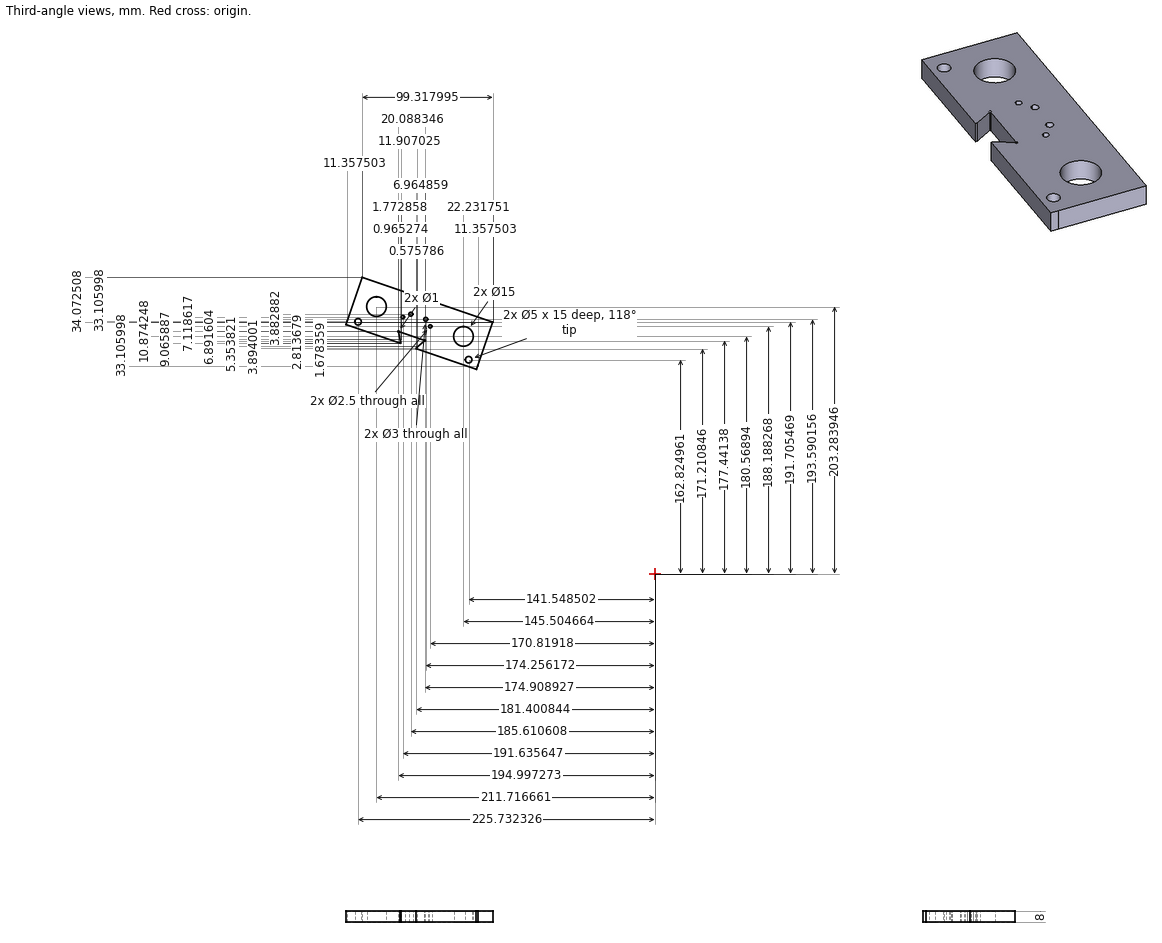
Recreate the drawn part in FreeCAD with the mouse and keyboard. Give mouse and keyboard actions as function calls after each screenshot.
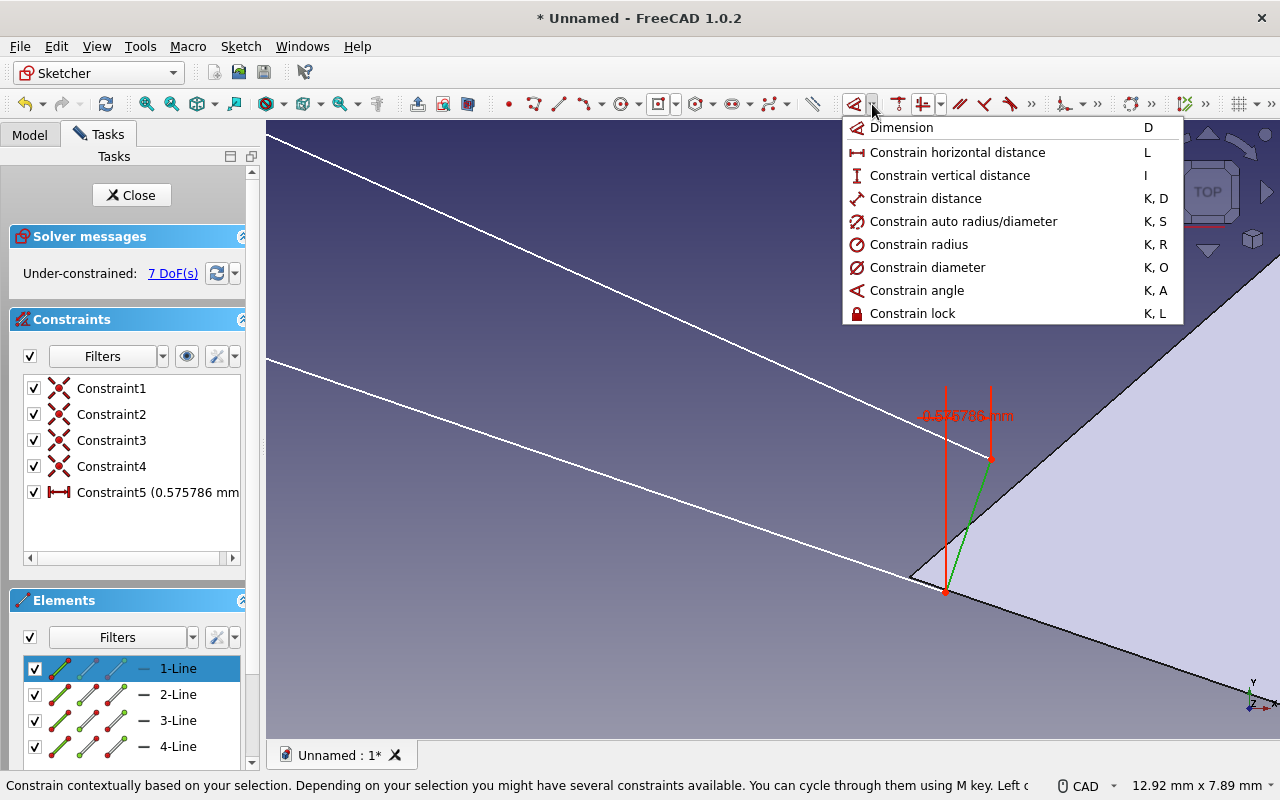
click(1013, 176)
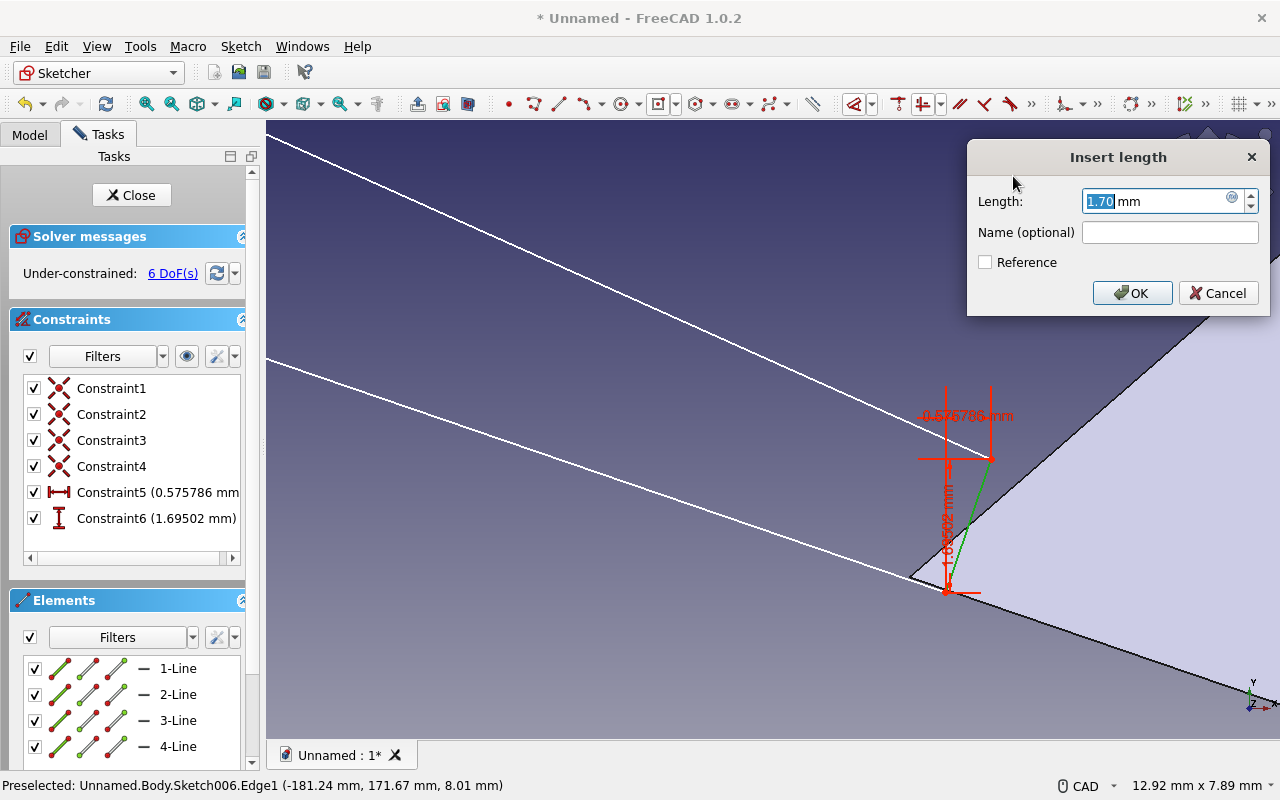
text(1.678359)
key(Return)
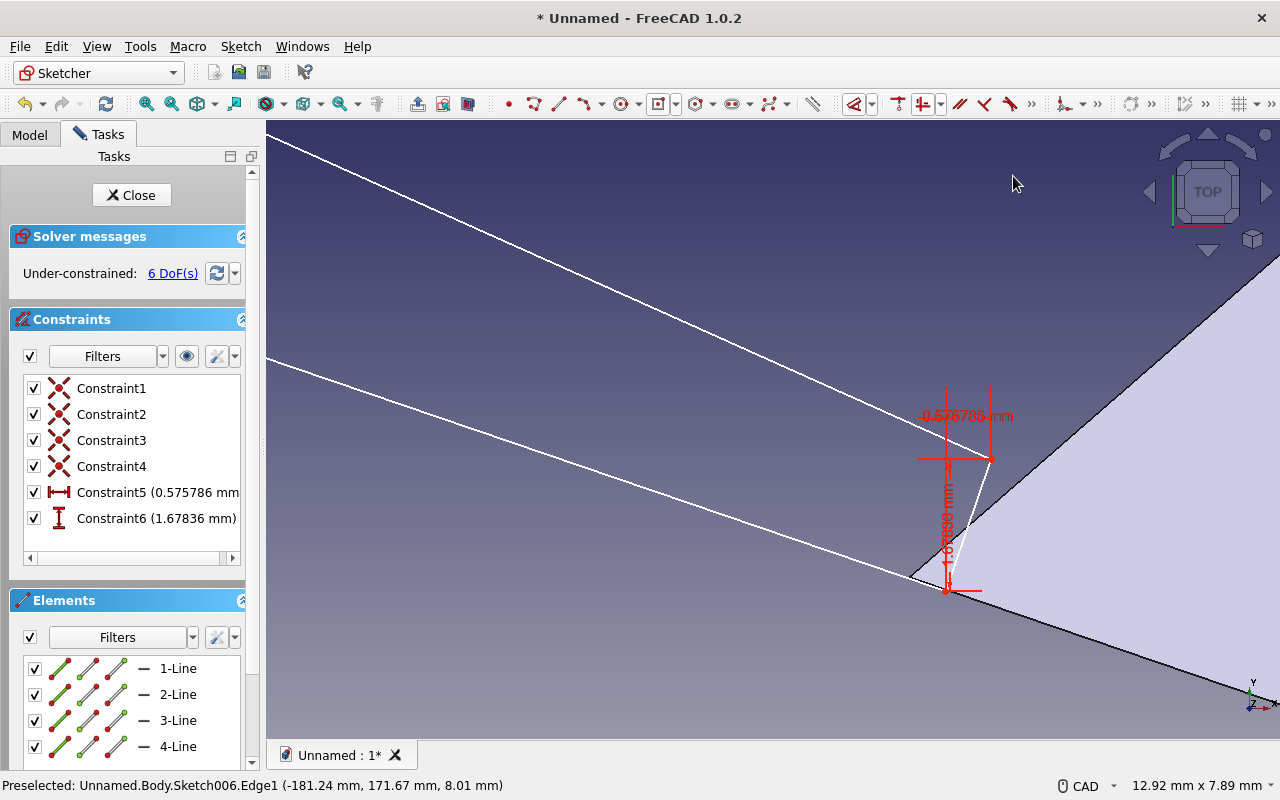
click(711, 334)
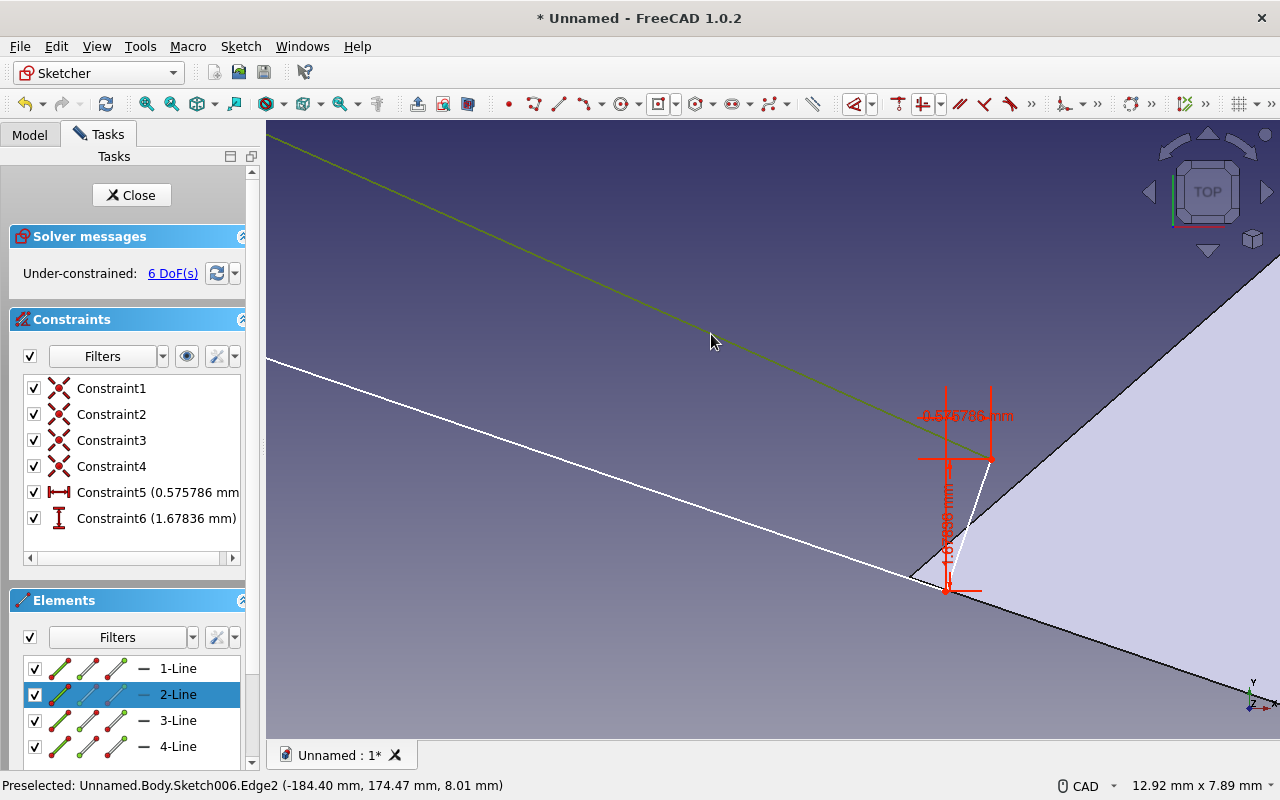
click(872, 104)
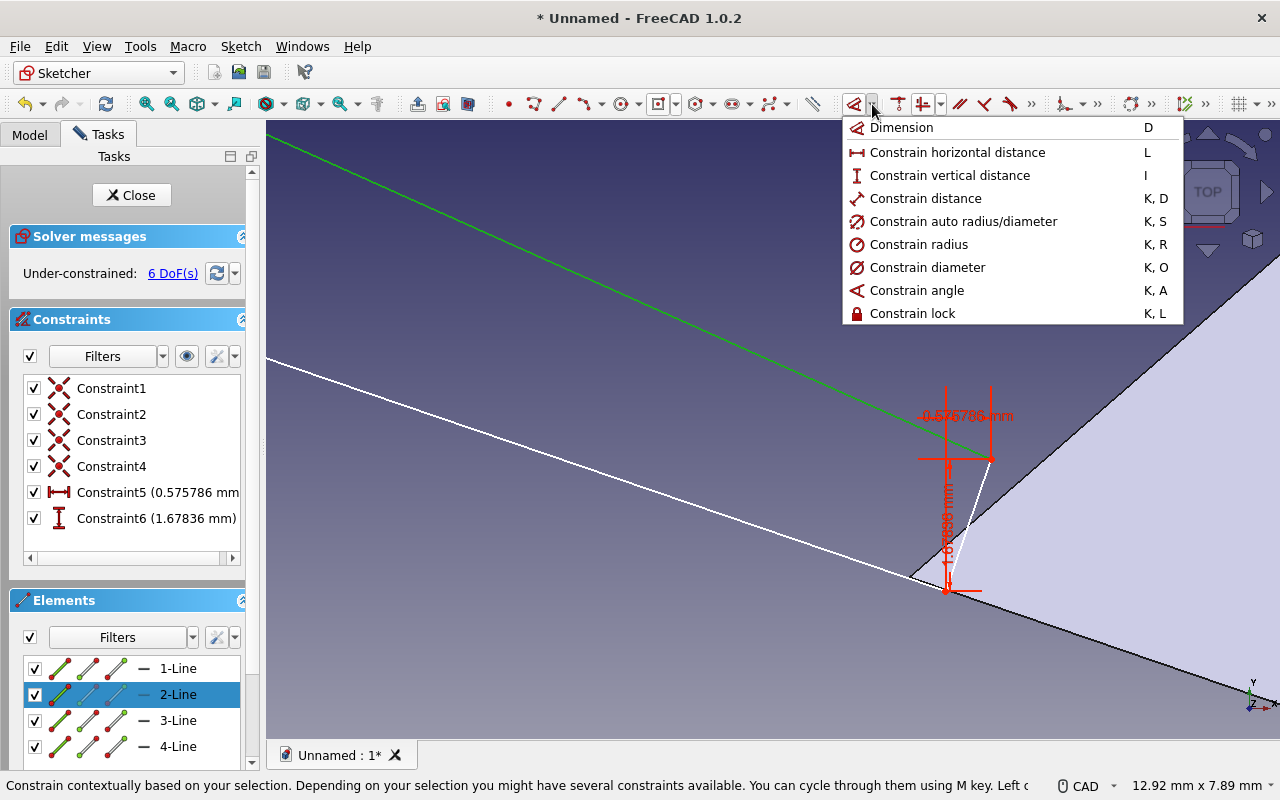
click(1013, 176)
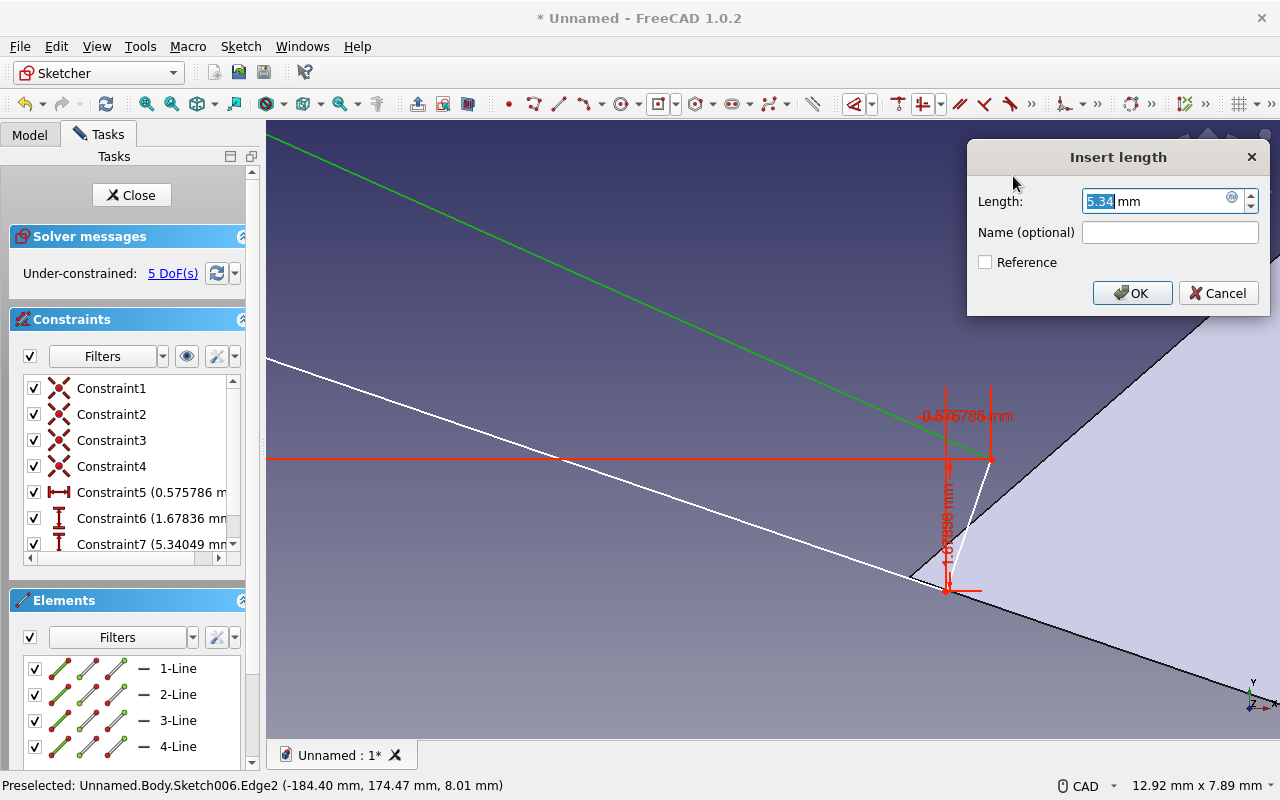
text(5.353821)
key(Return)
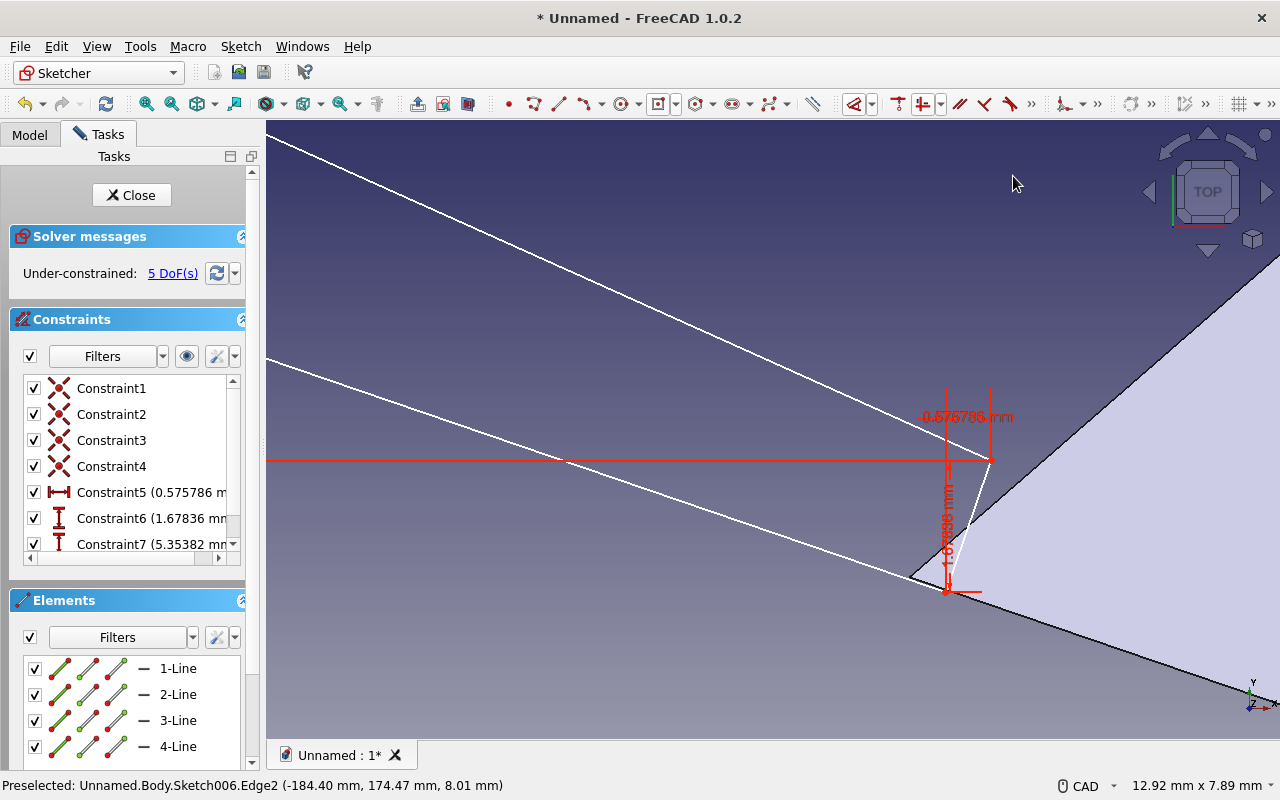
scroll(969, 570, down, 3)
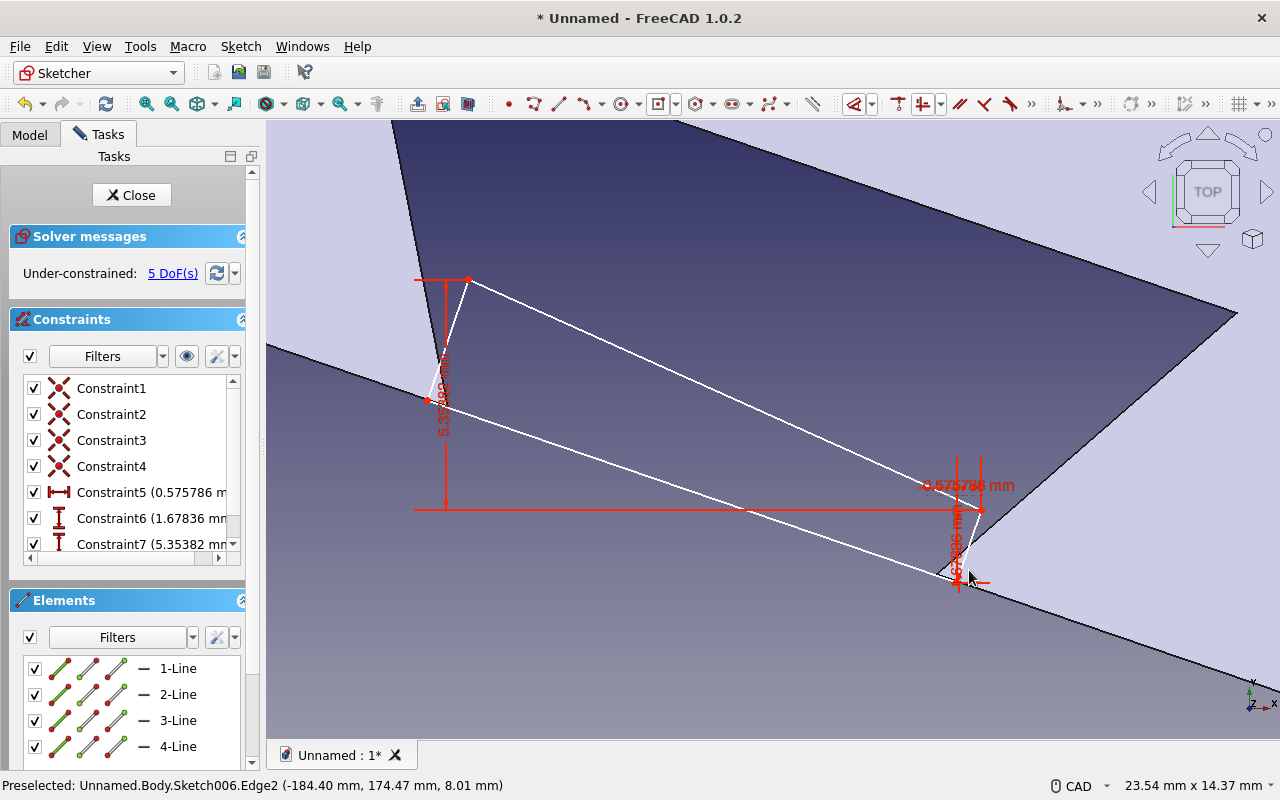
click(456, 316)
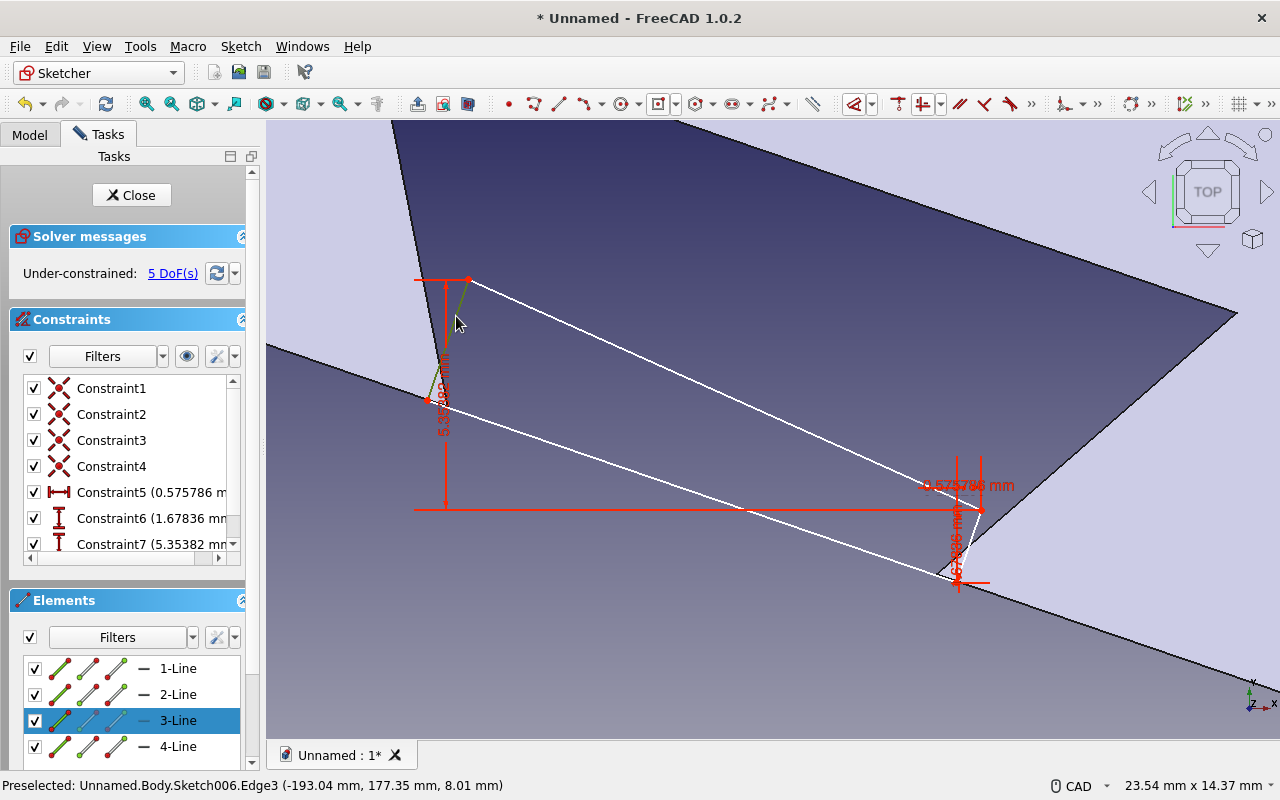
key(l)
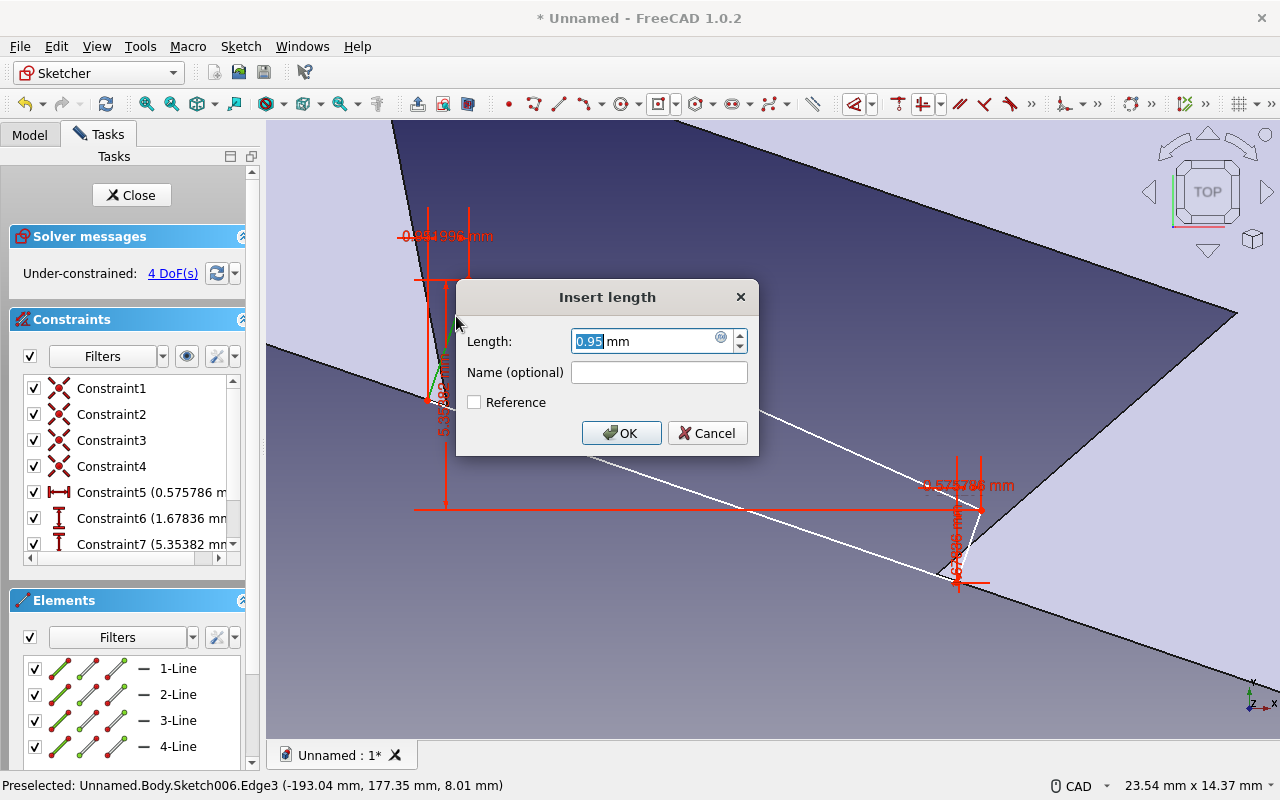
text(0.965274)
key(Return)